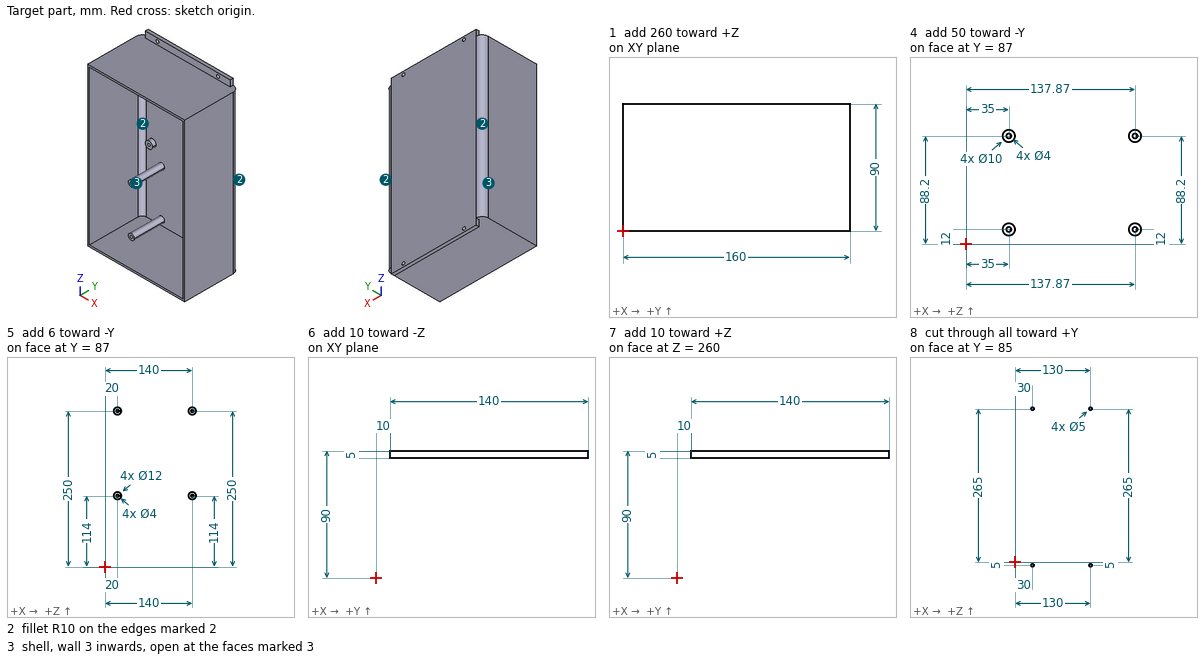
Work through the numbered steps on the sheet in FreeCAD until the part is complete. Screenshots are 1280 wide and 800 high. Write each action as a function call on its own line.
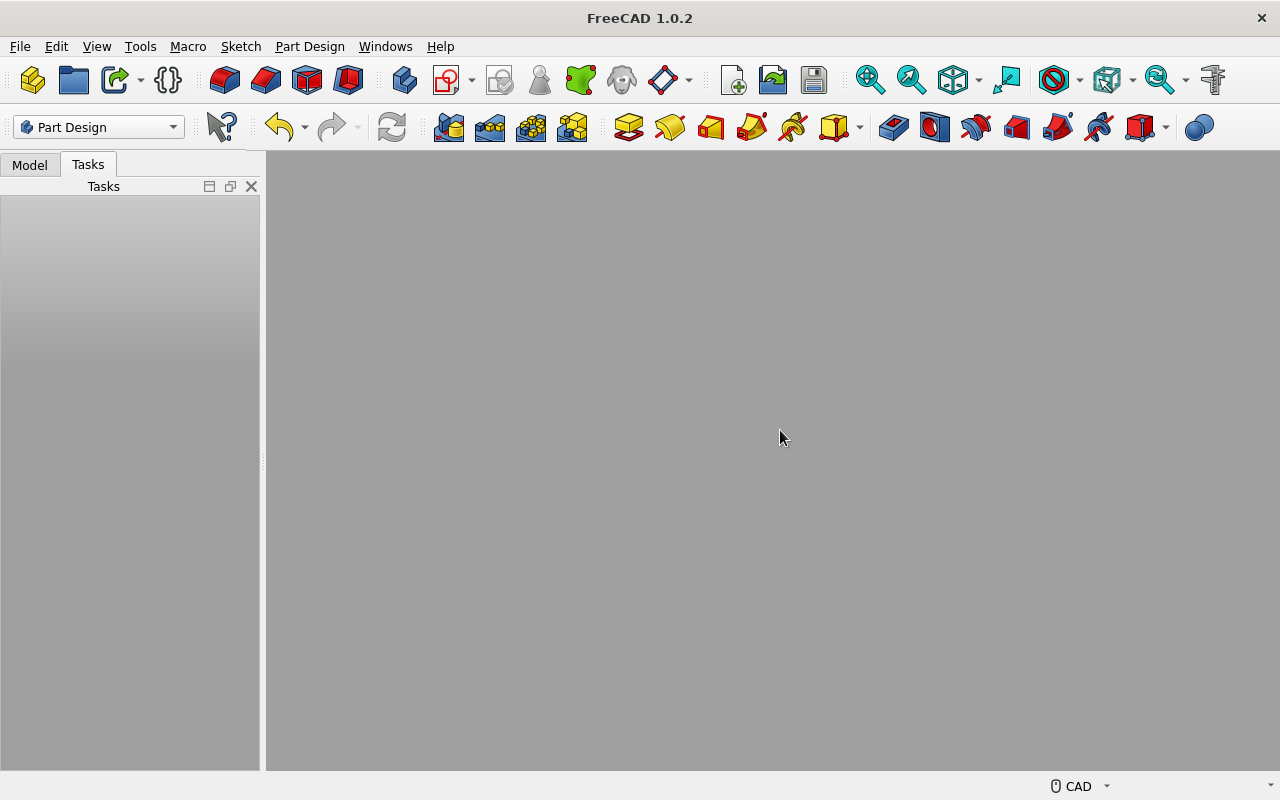
click(732, 80)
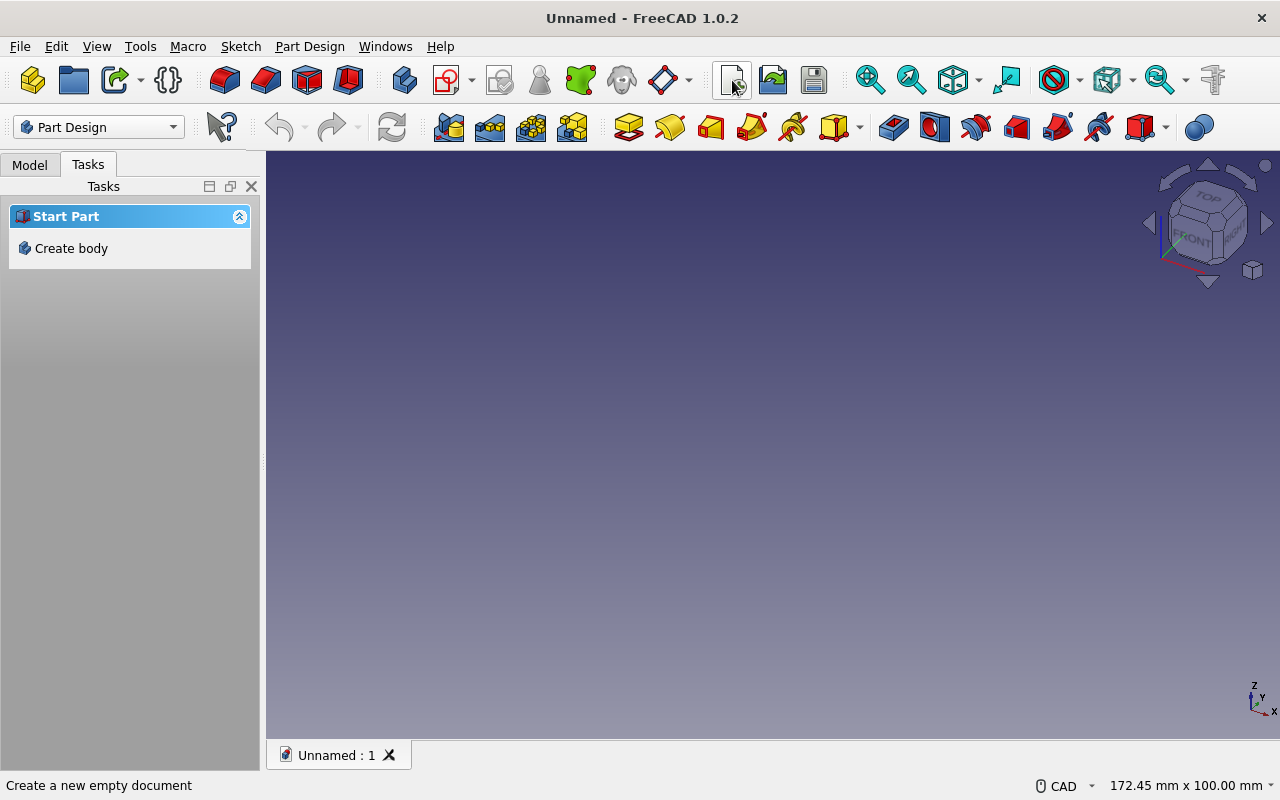
click(446, 80)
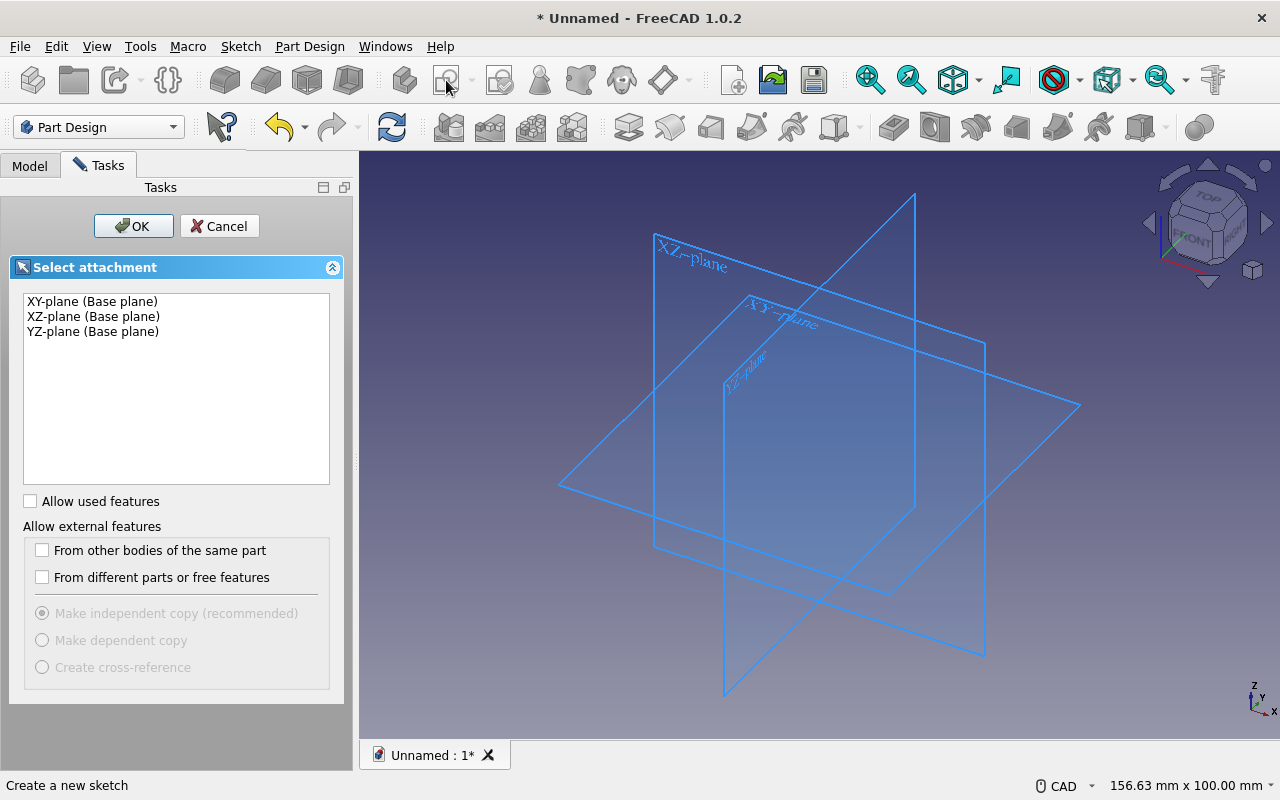
click(84, 302)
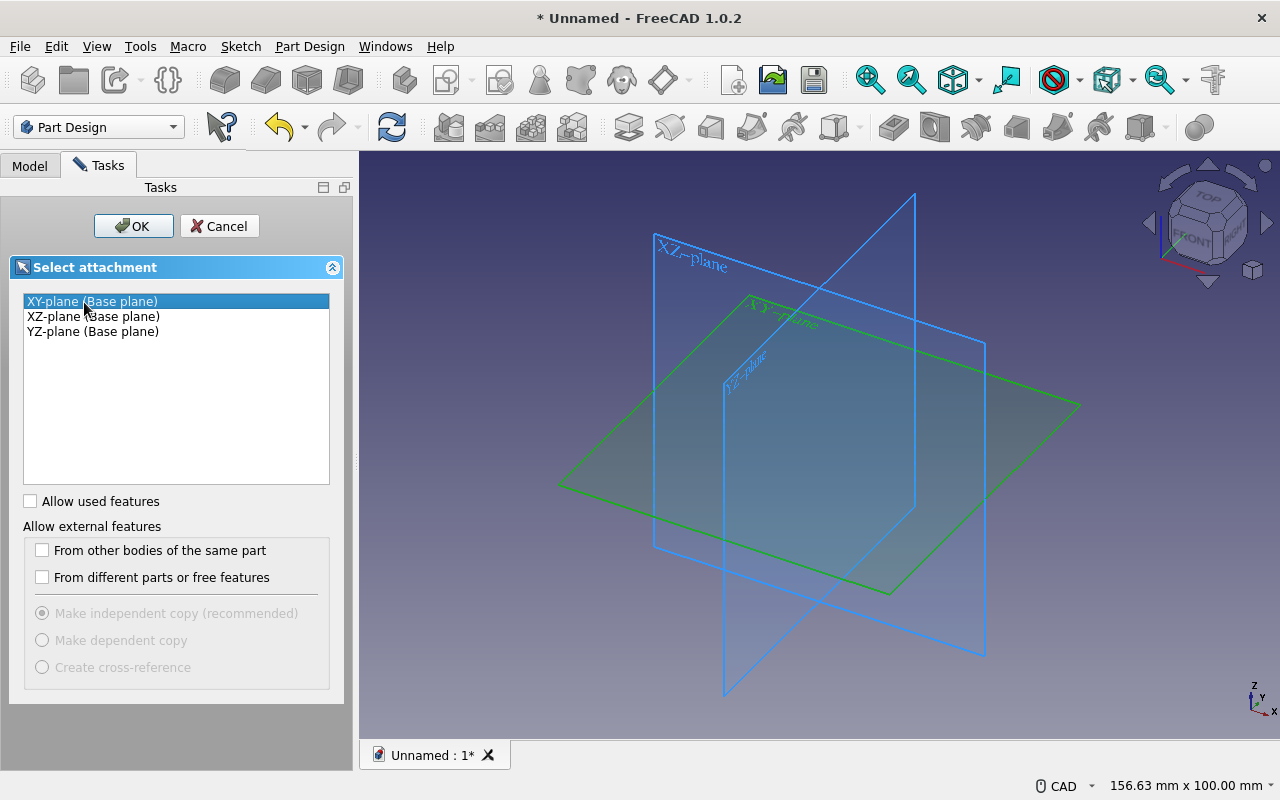
click(134, 226)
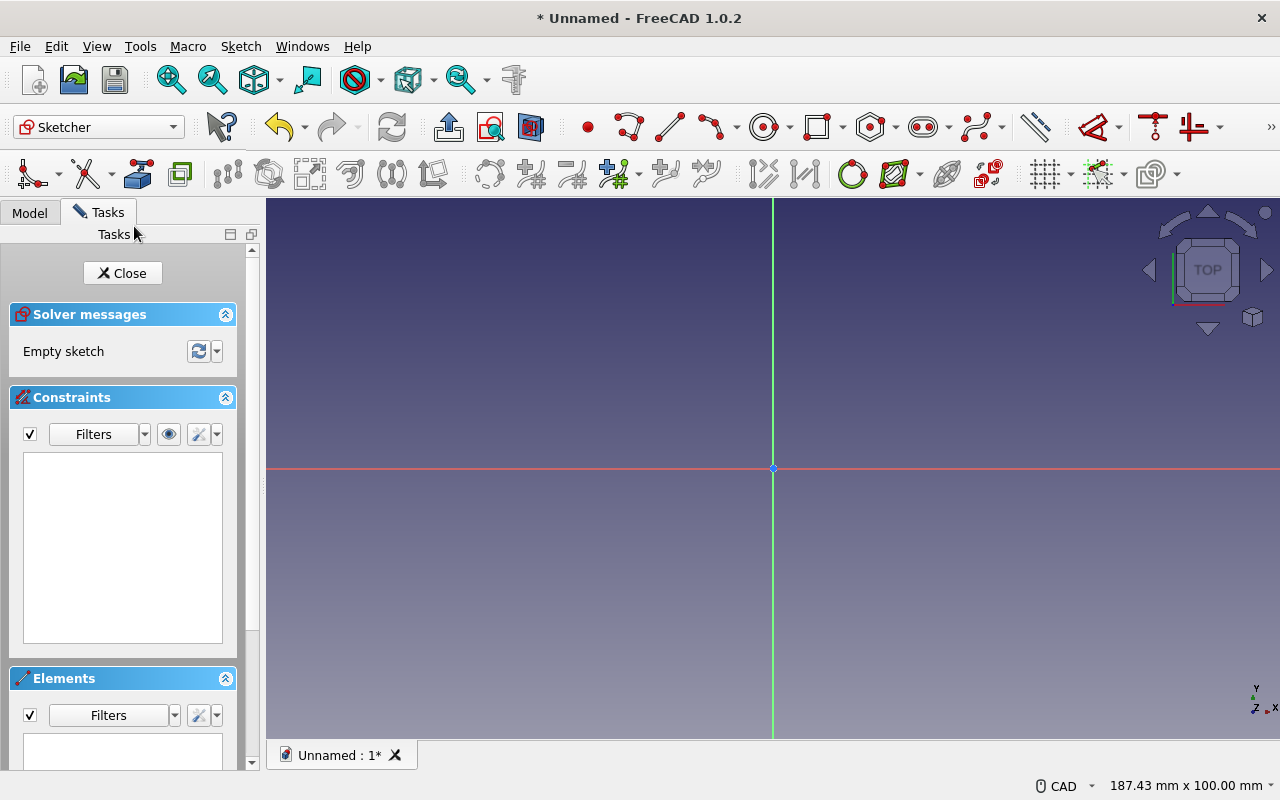
scroll(294, 711, down, 3)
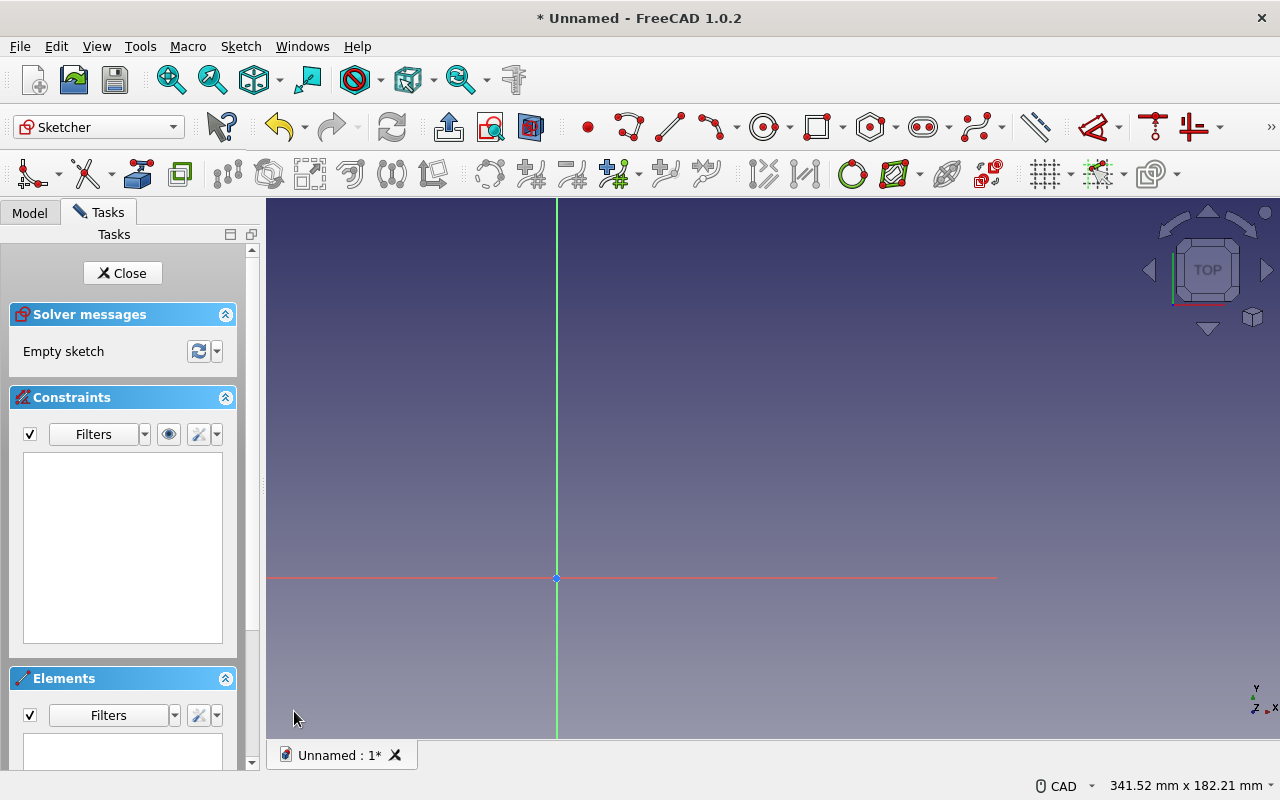
click(816, 128)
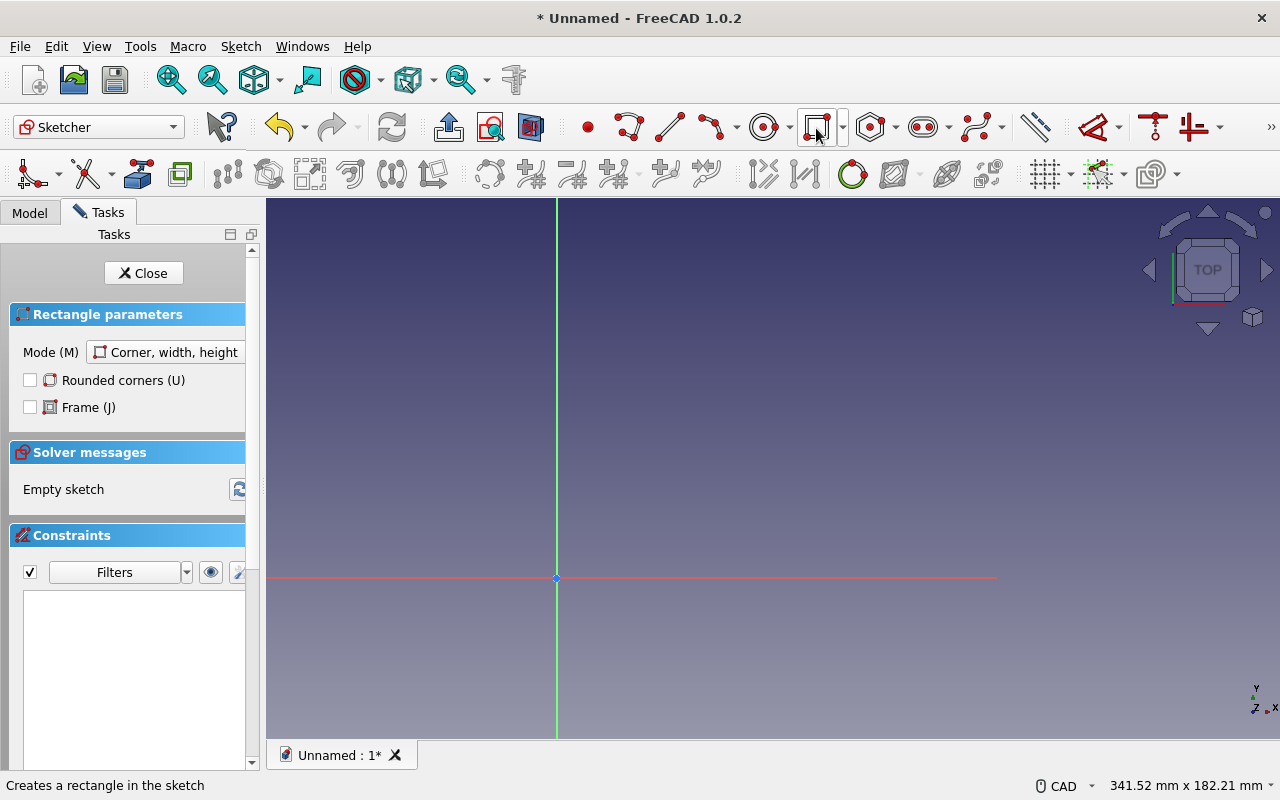
click(557, 578)
click(1032, 311)
key(Escape)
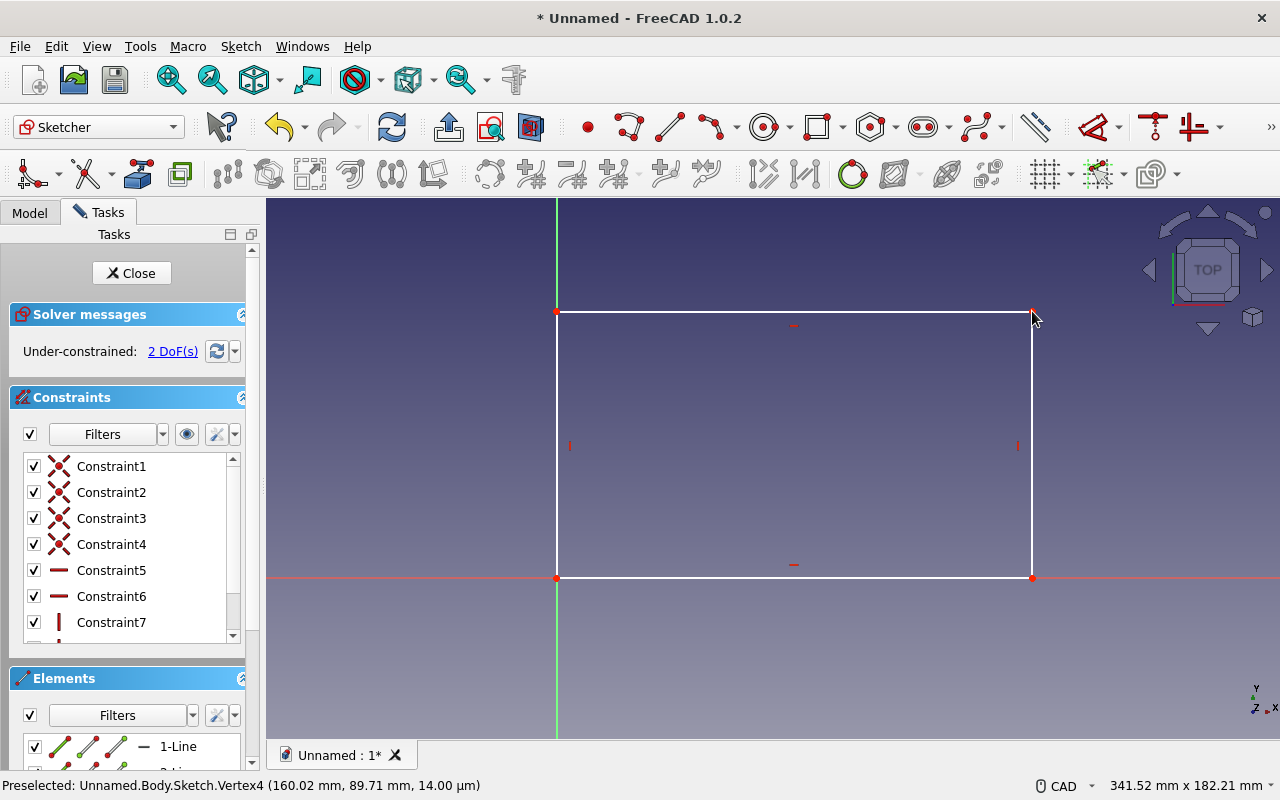
key(d)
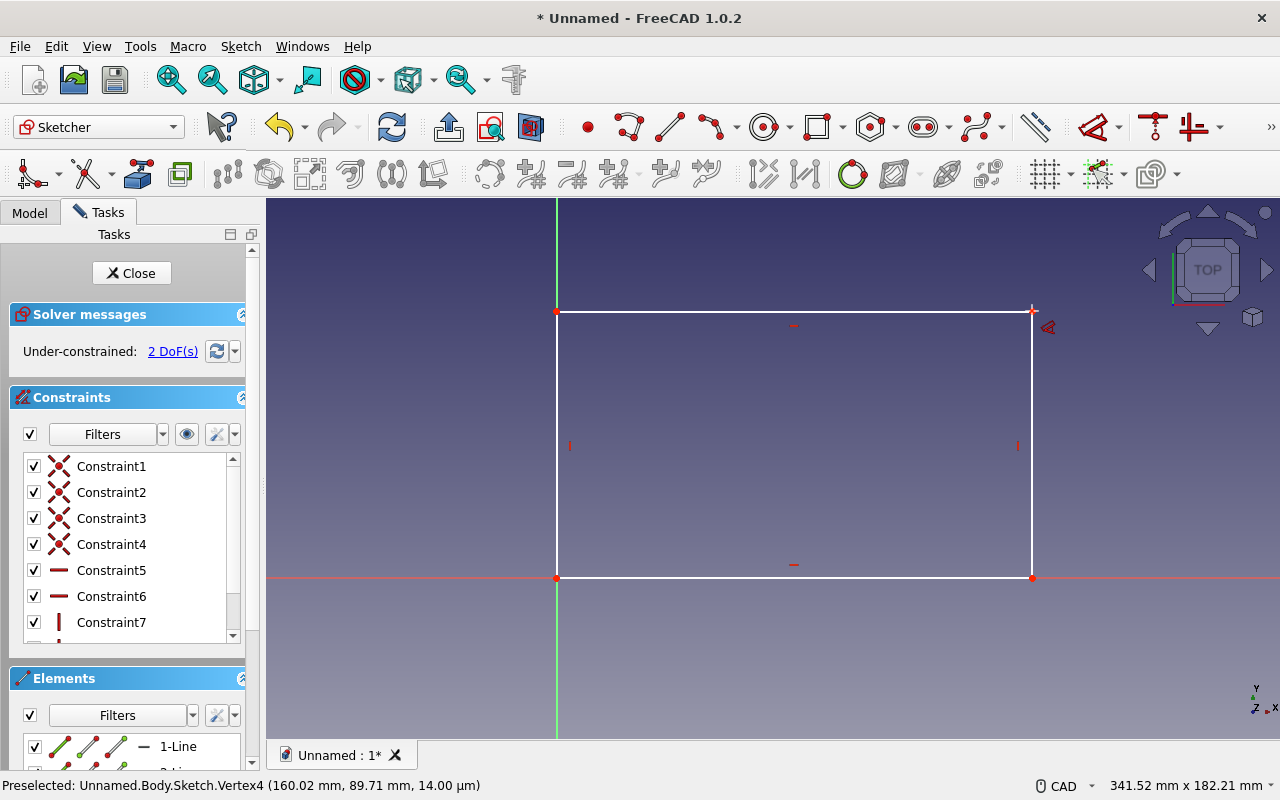
click(1032, 498)
click(1066, 445)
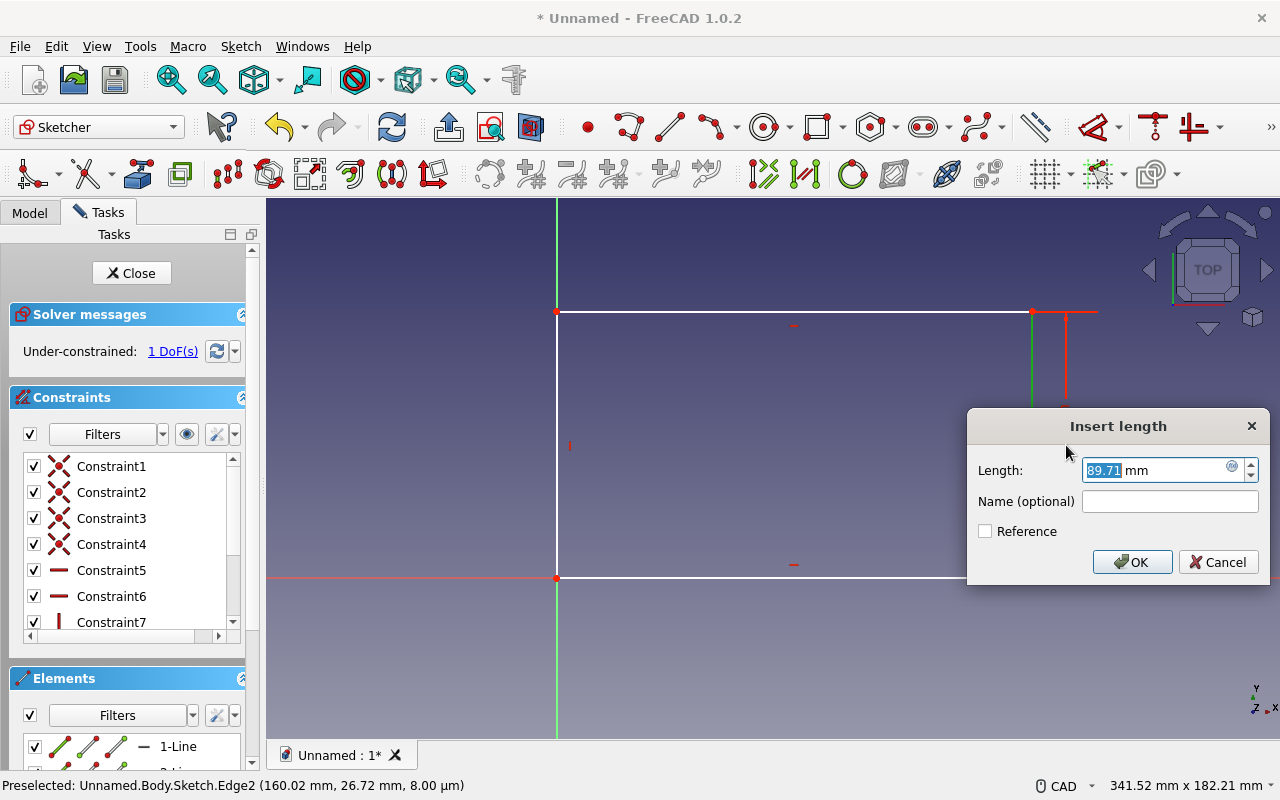
text(90)
key(Return)